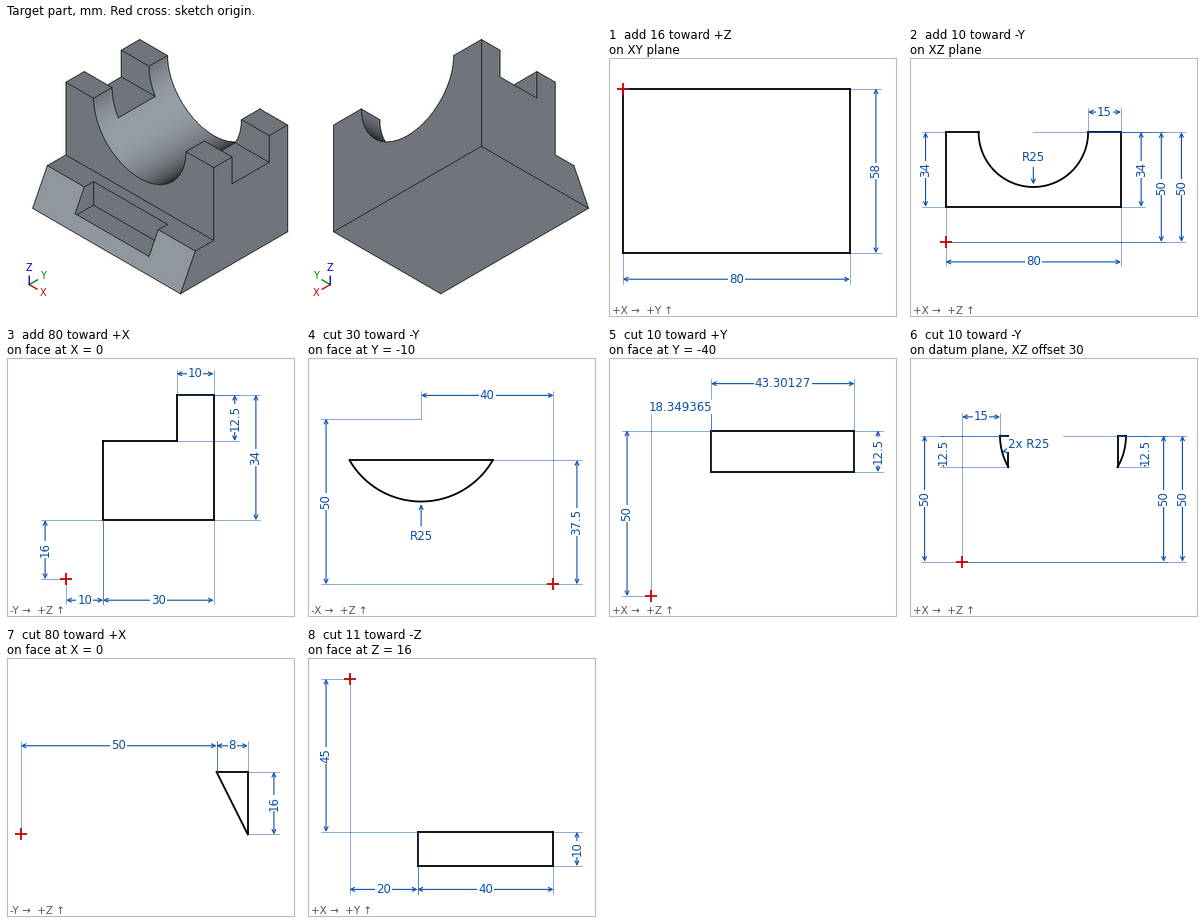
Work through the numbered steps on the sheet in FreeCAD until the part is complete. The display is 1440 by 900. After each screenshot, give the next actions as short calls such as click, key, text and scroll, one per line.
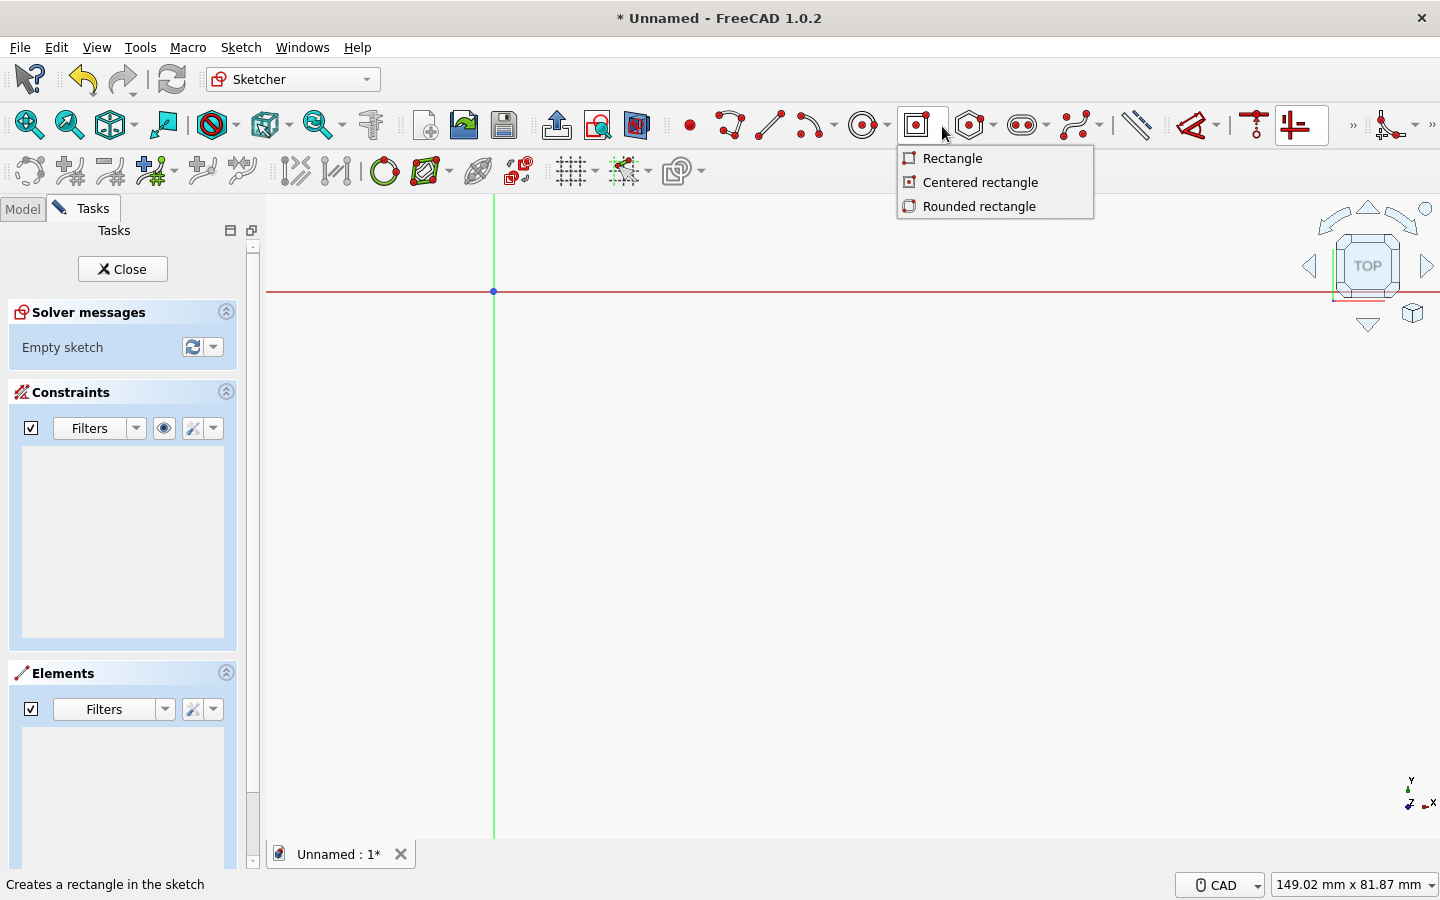
click(996, 158)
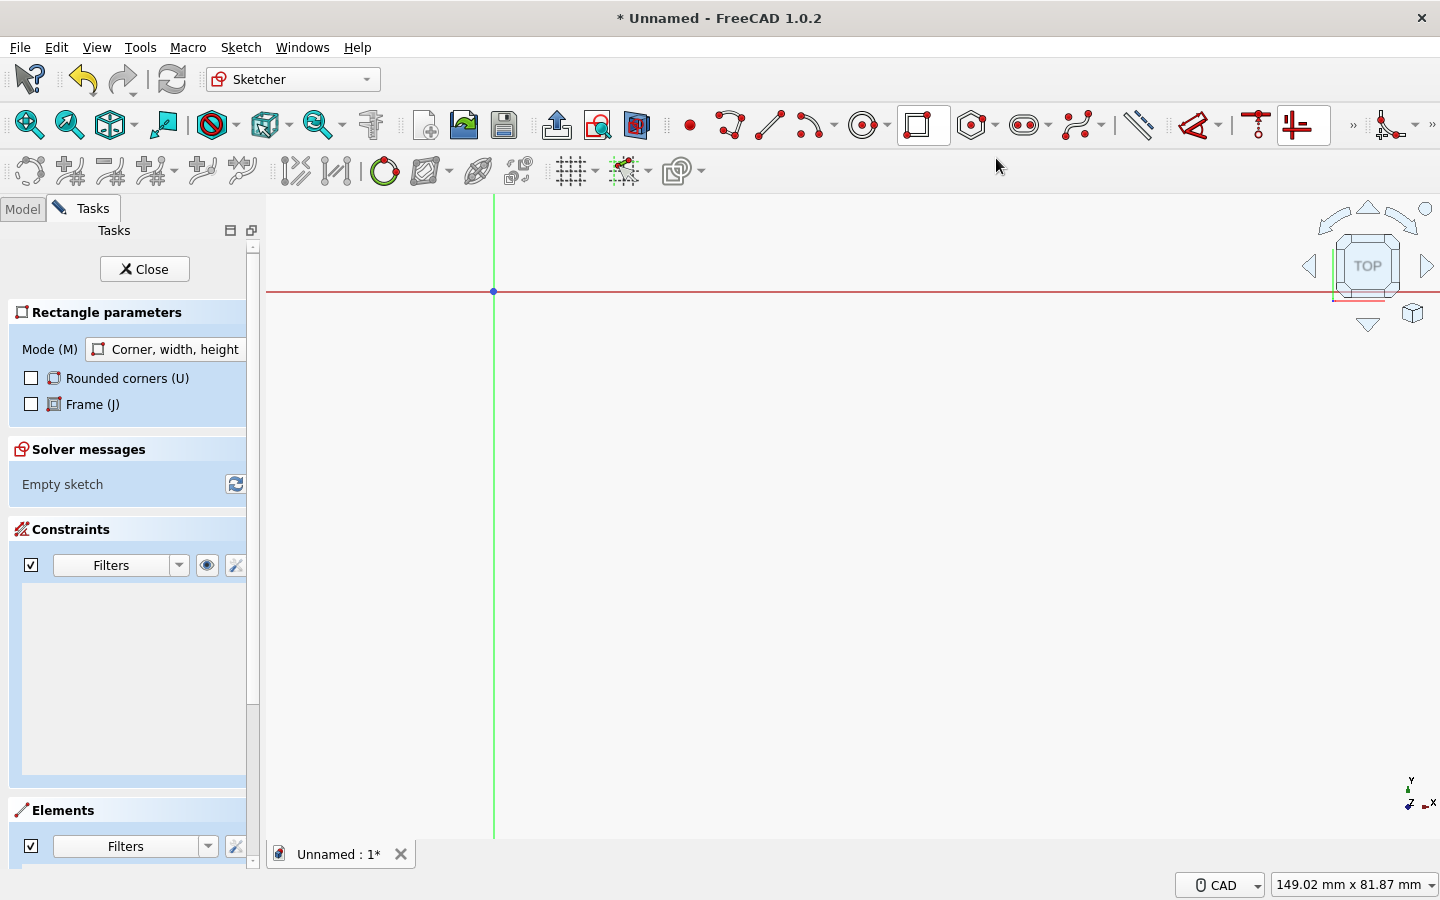
click(494, 292)
move(1124, 748)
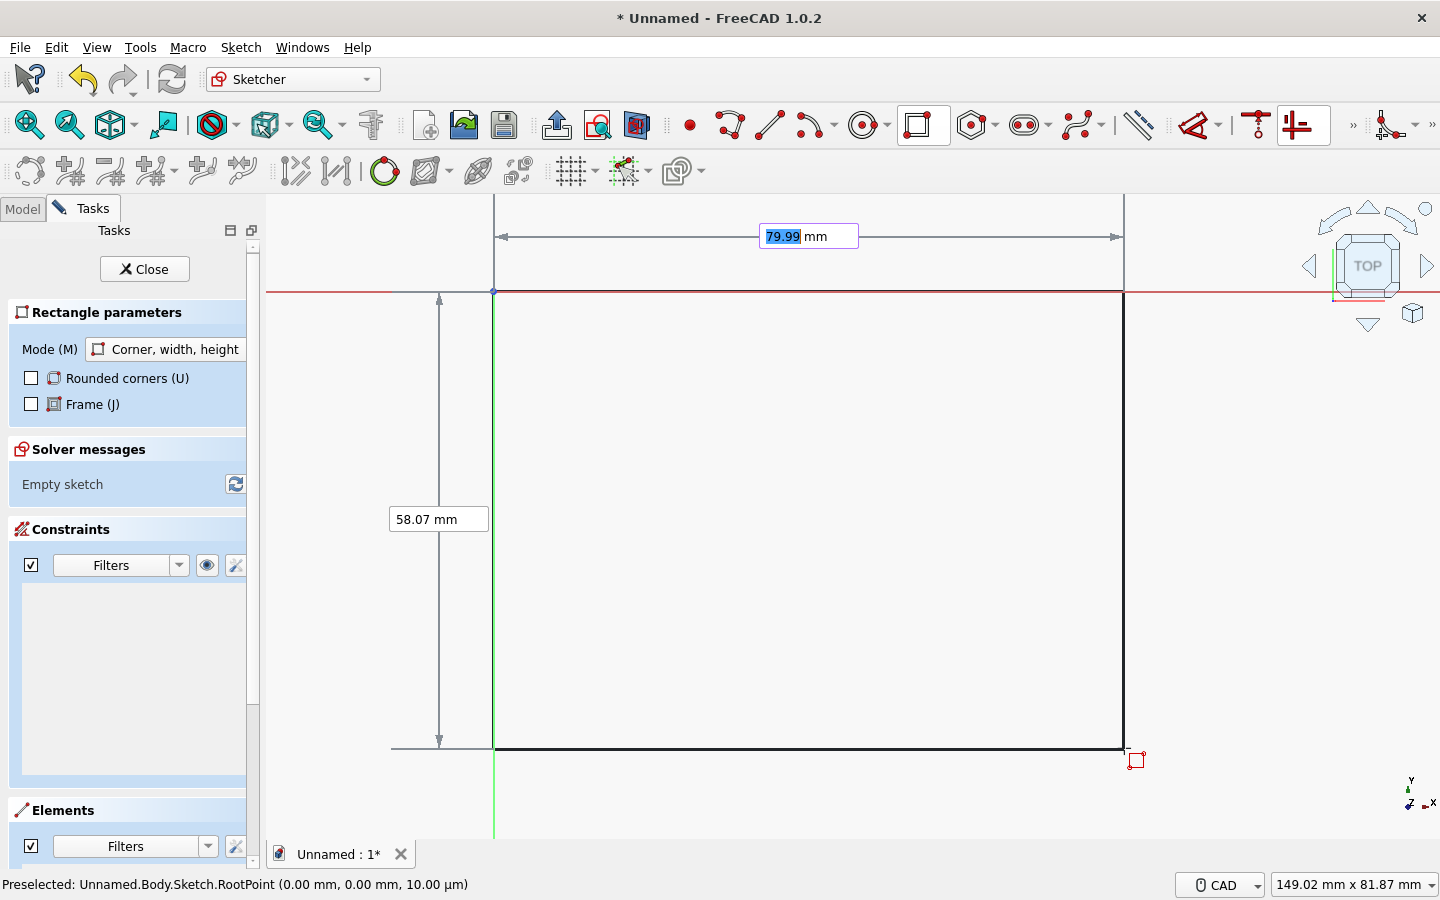
text(80)
key(Tab)
text(58)
key(Return)
key(Escape)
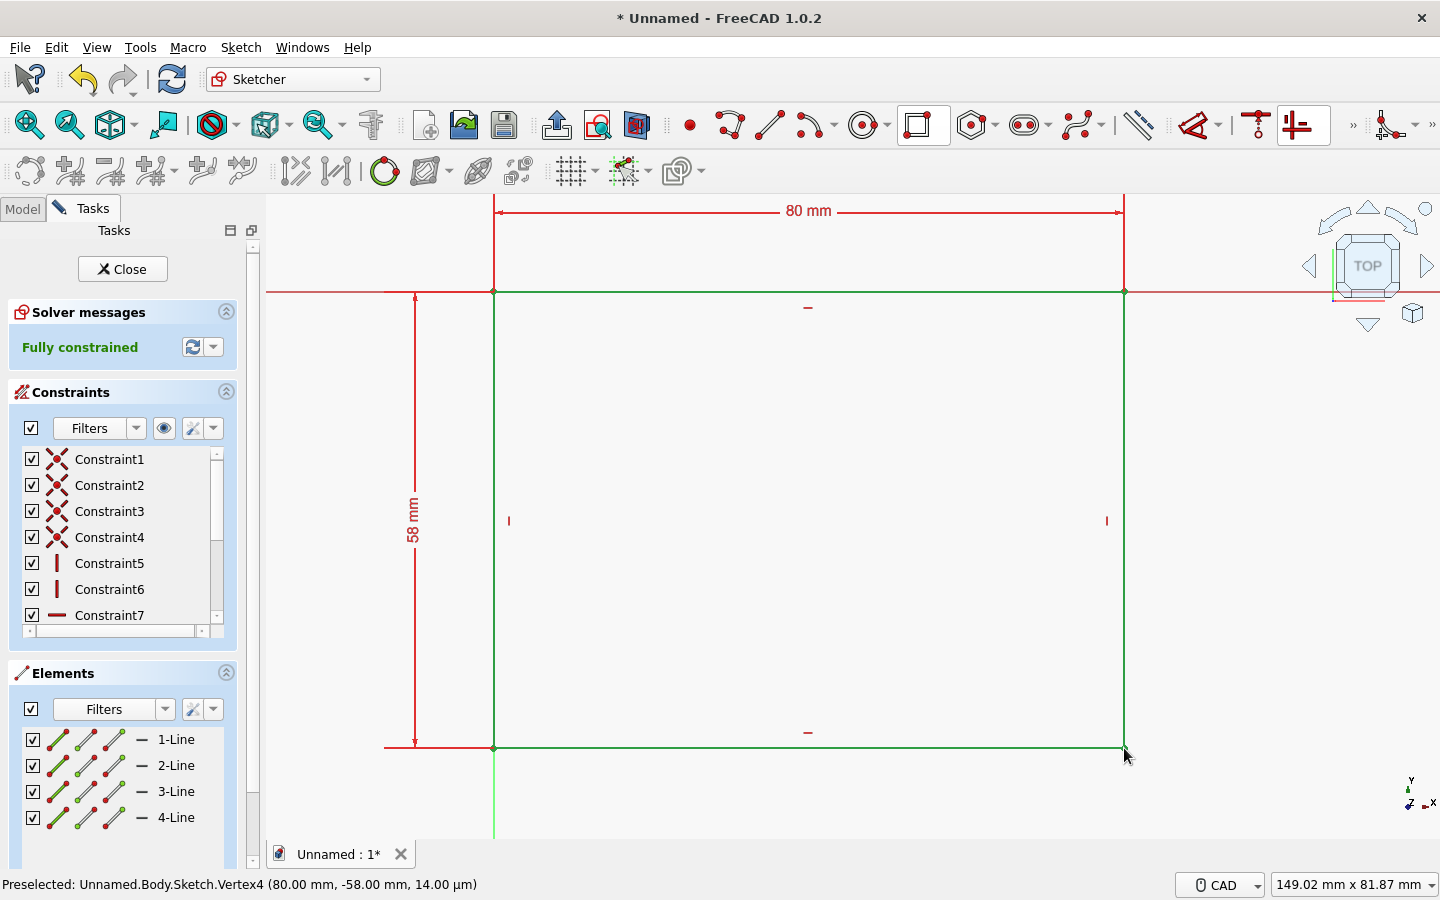
click(123, 269)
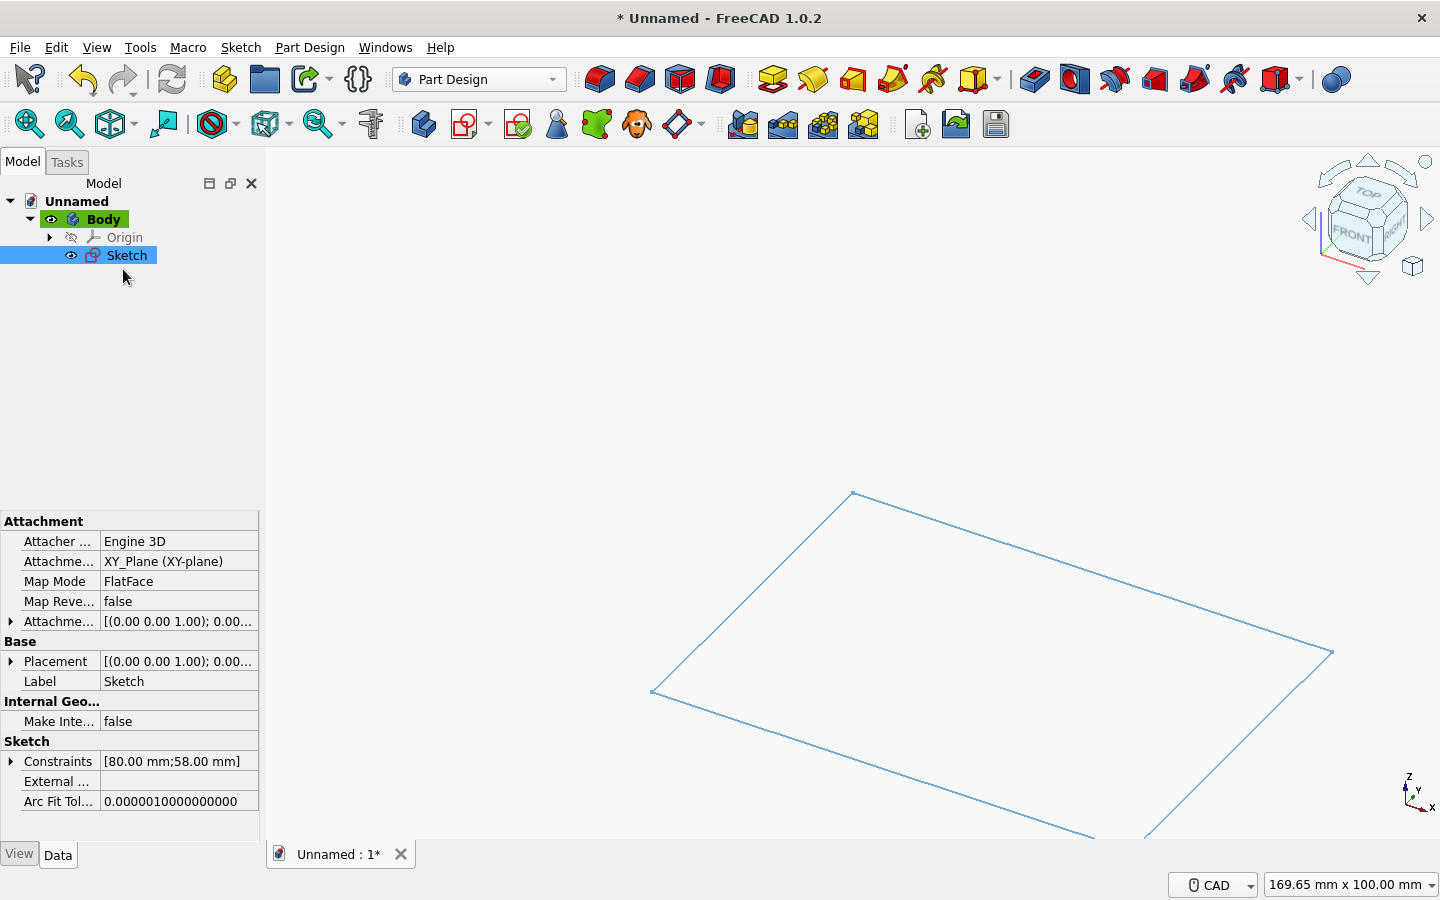
click(774, 80)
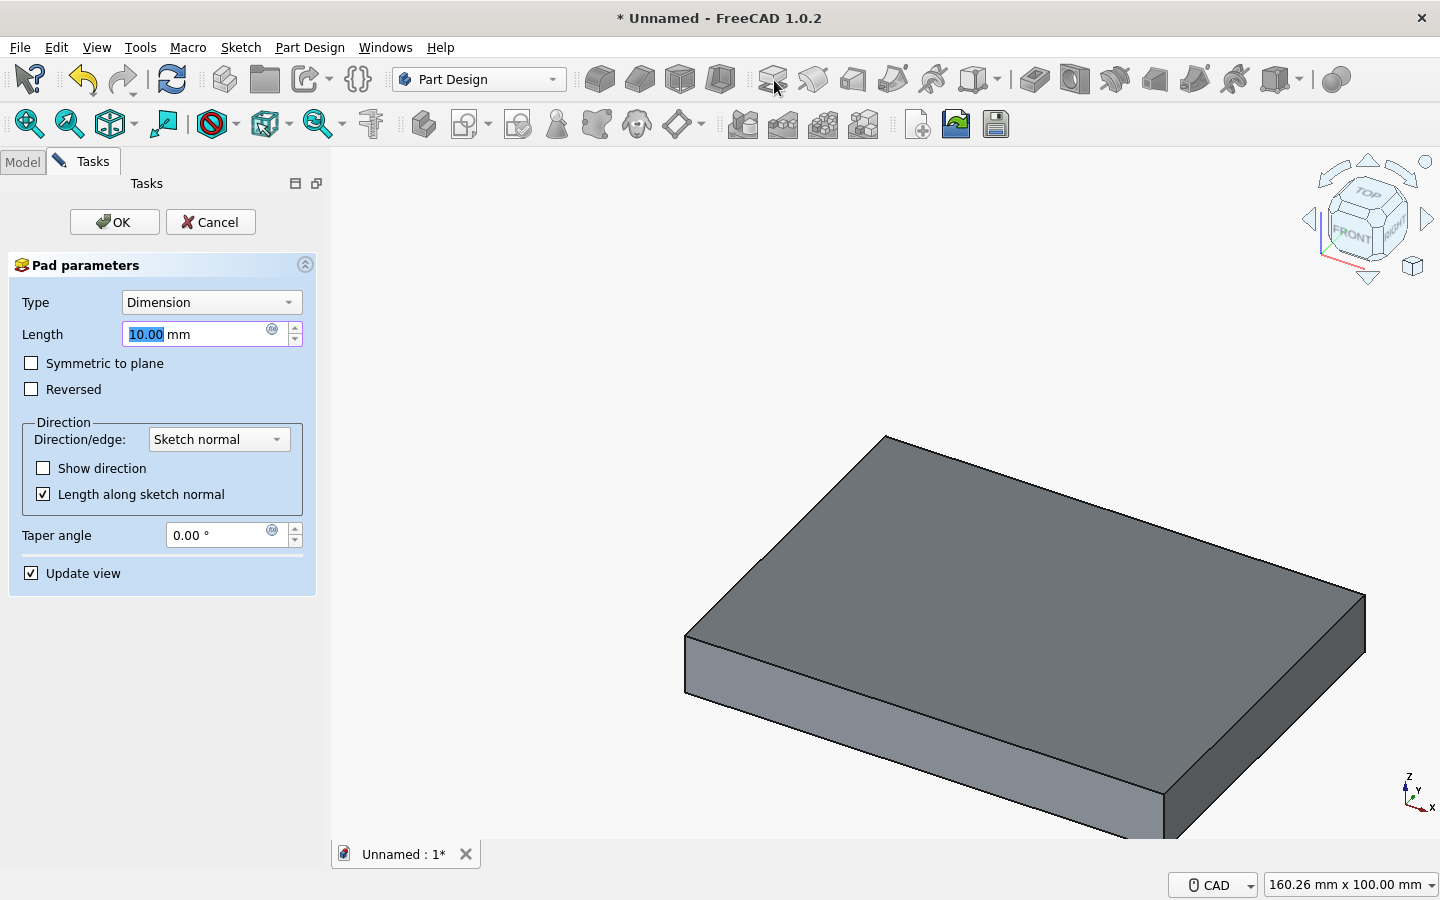
text(16)
key(Tab)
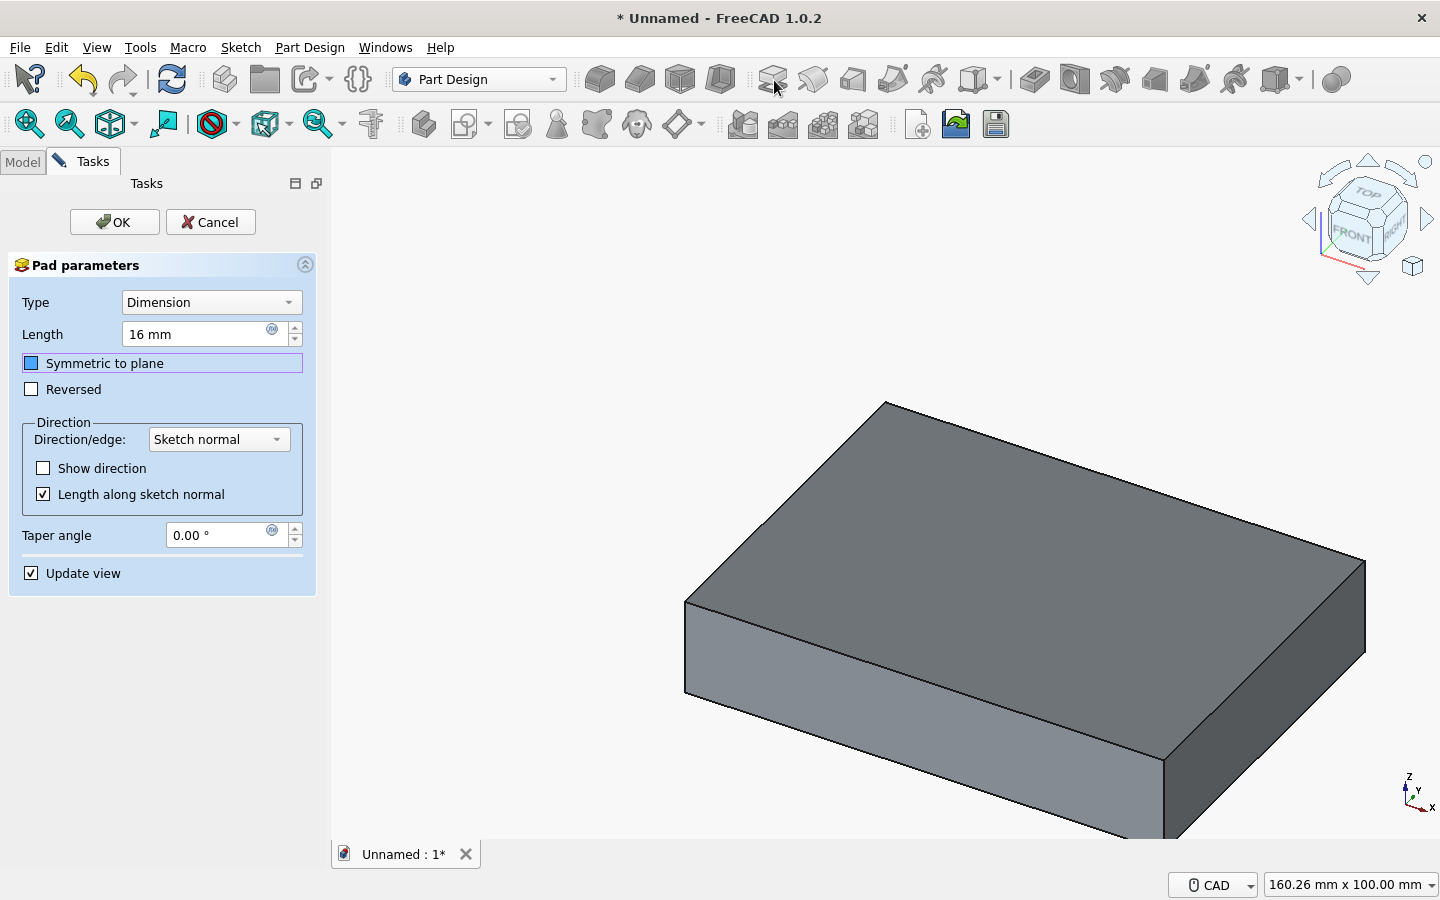
click(115, 222)